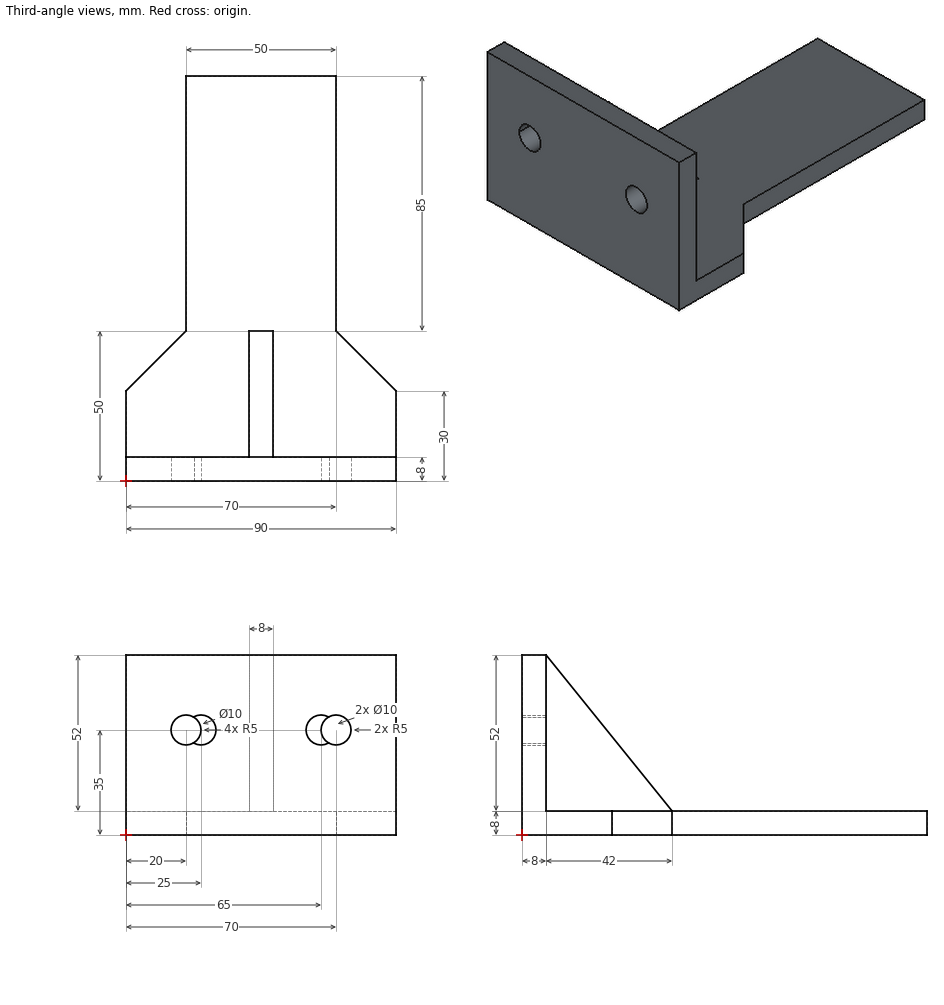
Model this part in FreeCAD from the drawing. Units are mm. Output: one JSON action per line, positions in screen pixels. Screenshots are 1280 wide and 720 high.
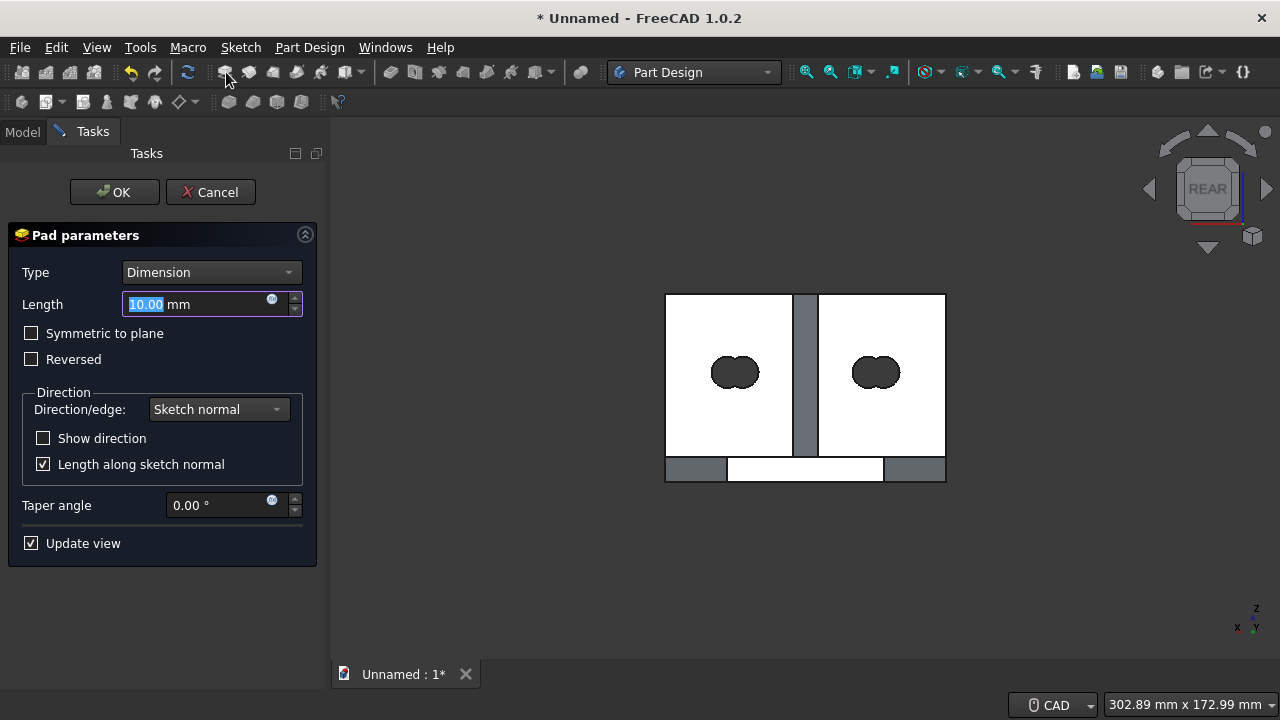
{"action": "type", "text": "8"}
{"action": "key", "text": "Tab"}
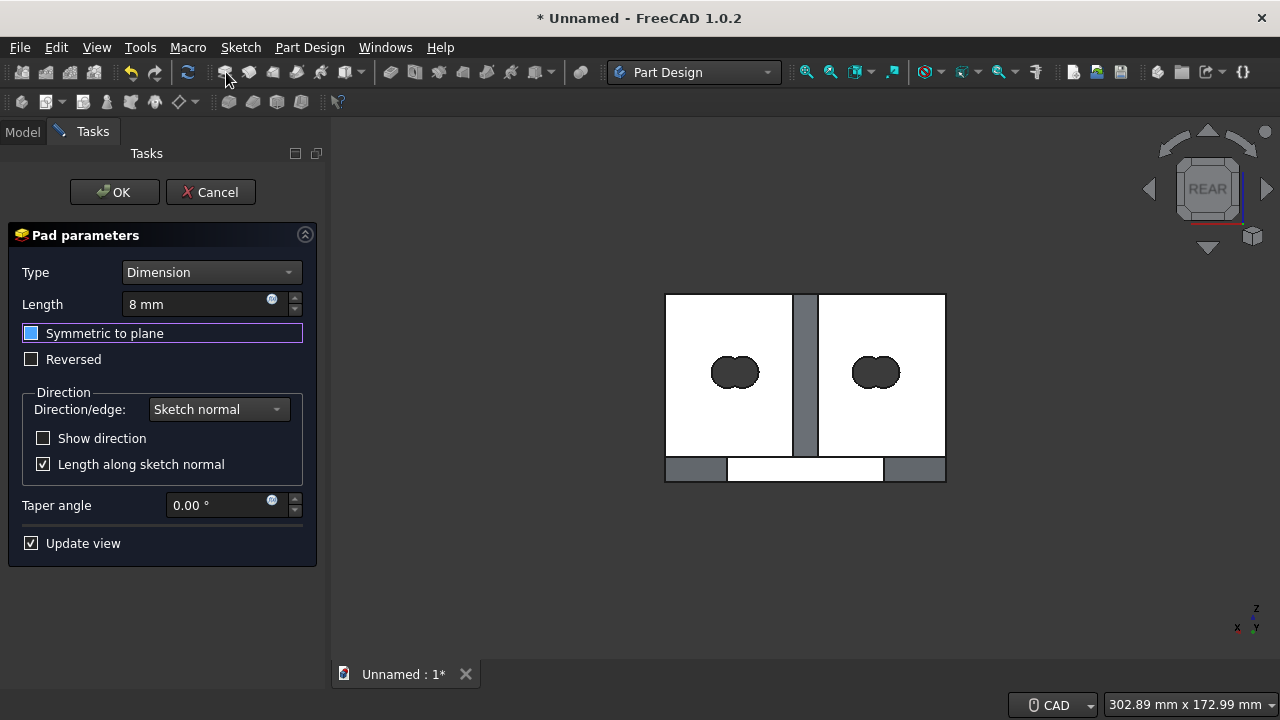
{"action": "left_click", "coordinate": [30, 359]}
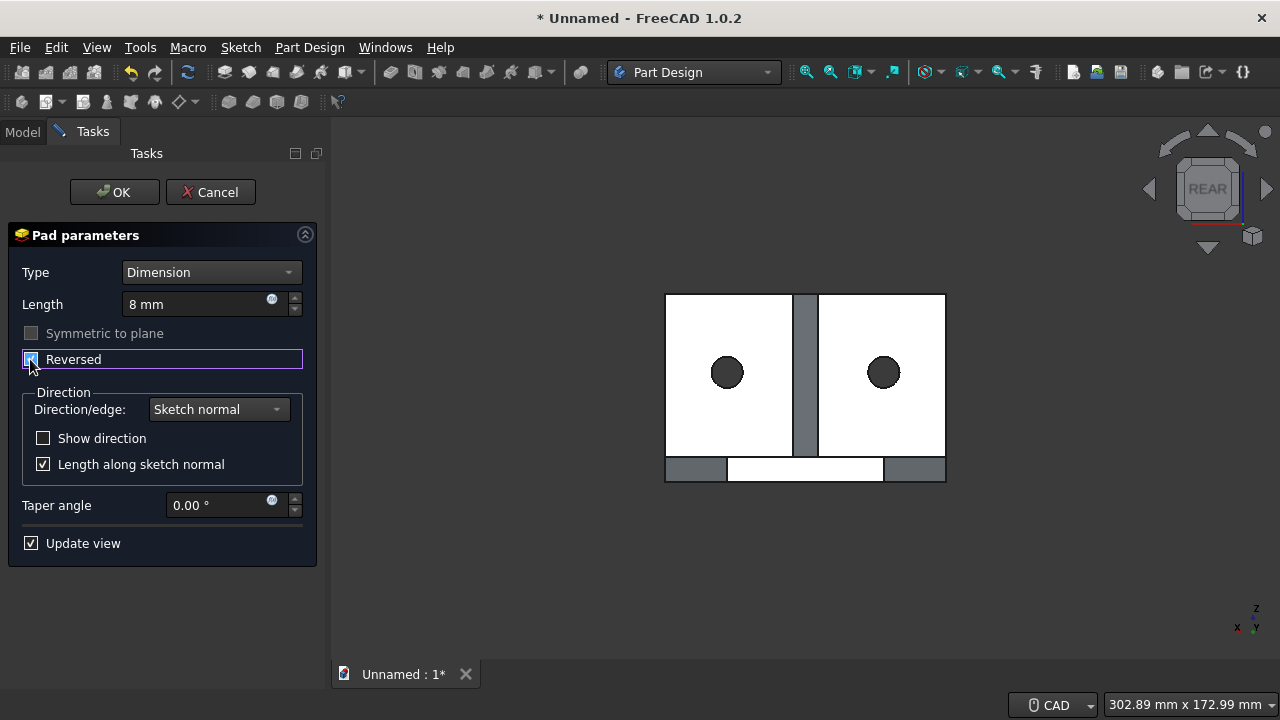
{"action": "left_click", "coordinate": [115, 192]}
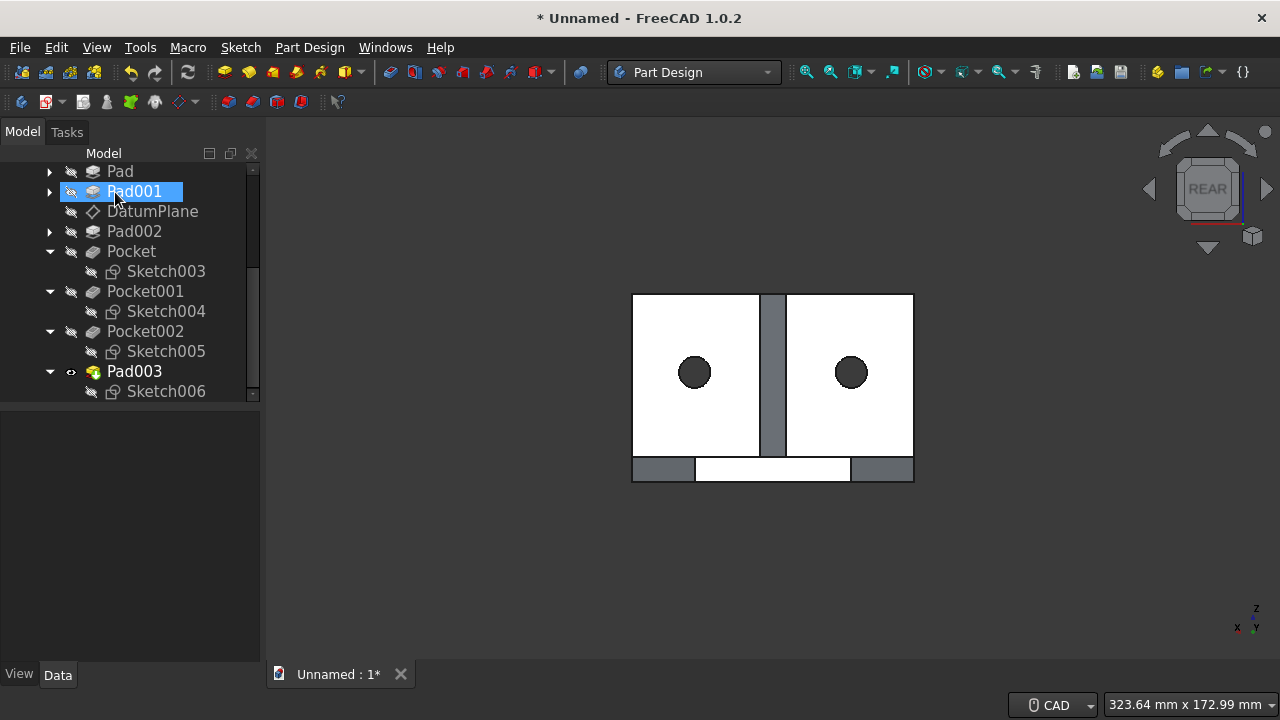
{"action": "key", "text": "0"}